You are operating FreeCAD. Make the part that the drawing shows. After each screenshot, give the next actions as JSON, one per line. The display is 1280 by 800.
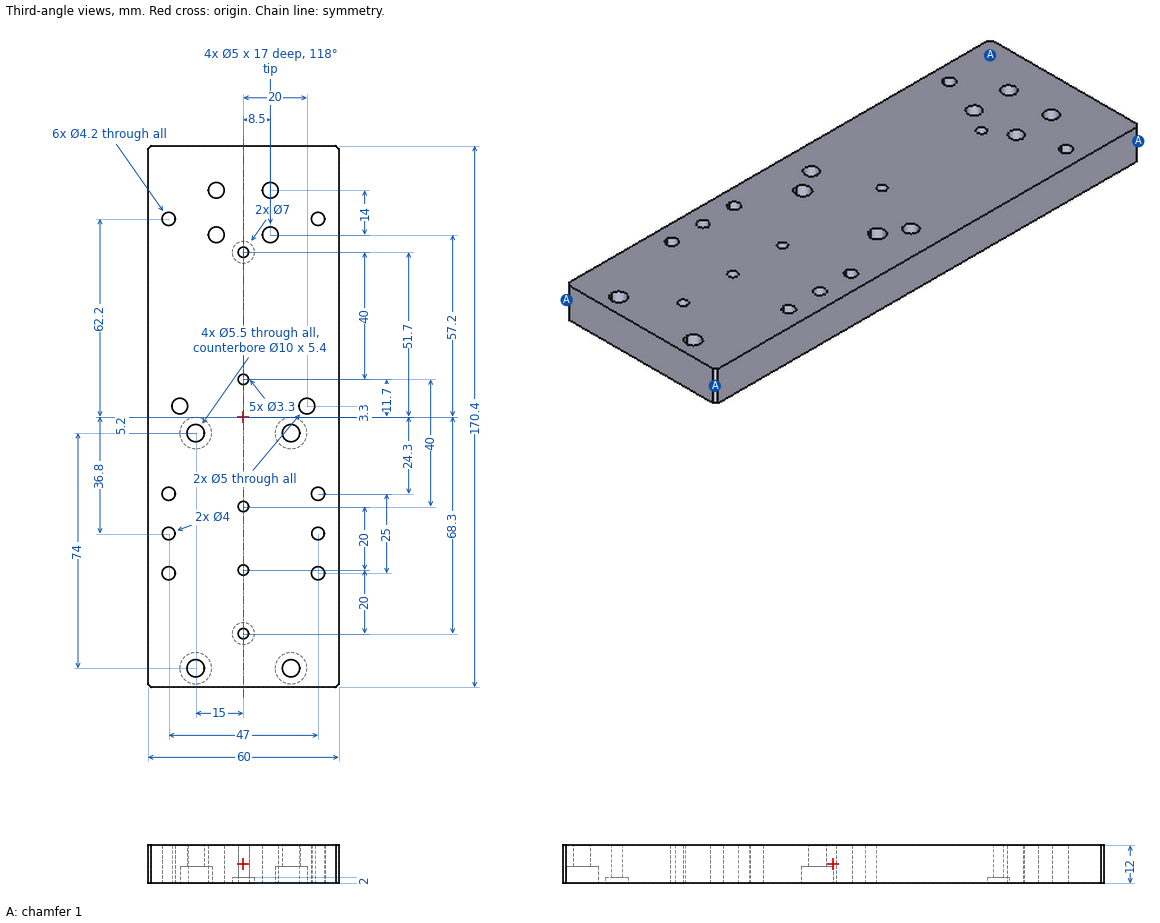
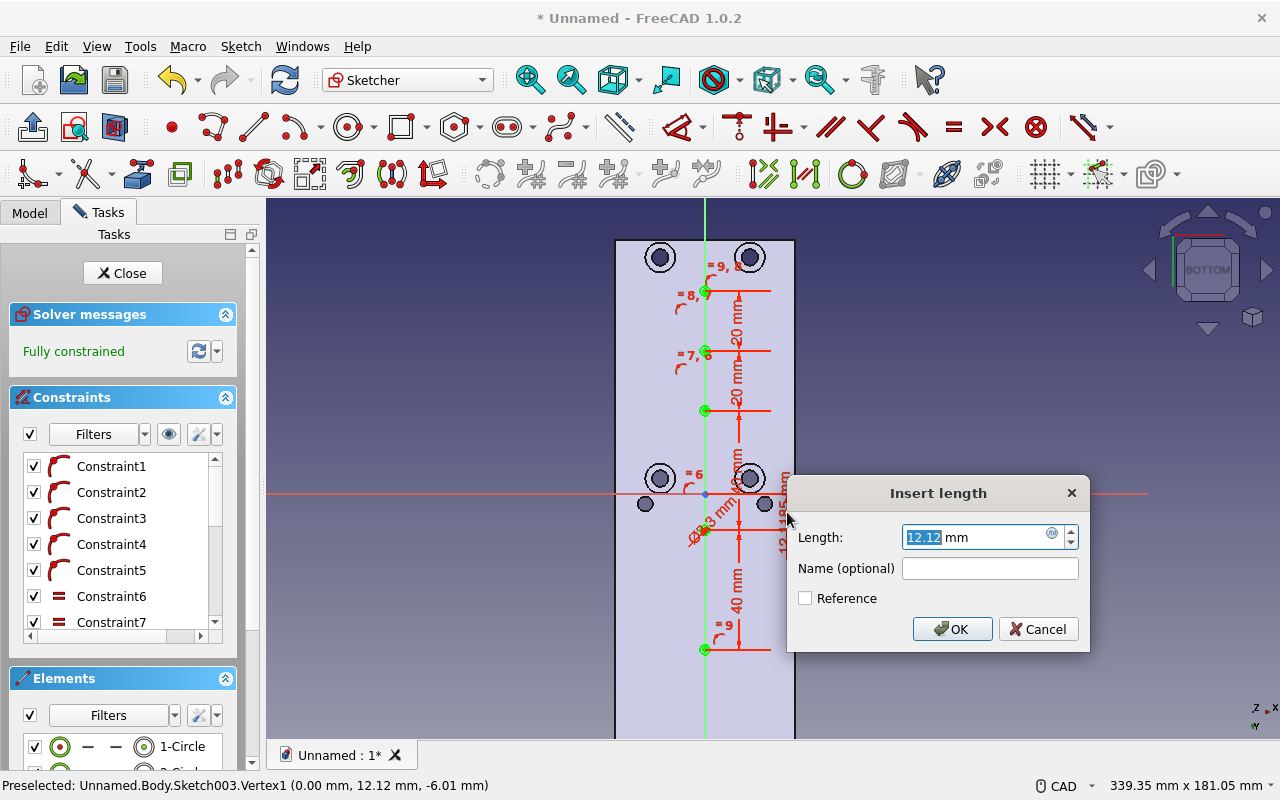
{"action": "type", "text": "11.7"}
{"action": "key", "text": "Return"}
{"action": "key", "text": "Escape"}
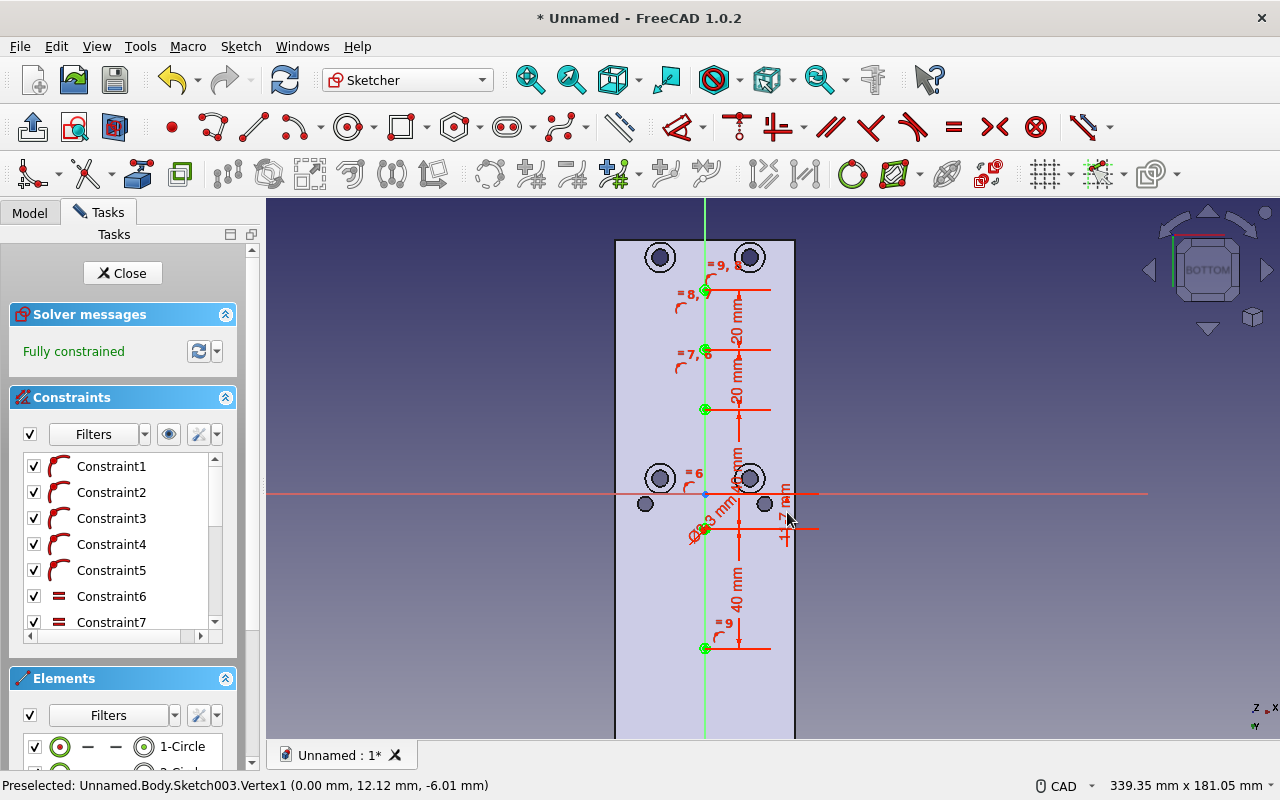
{"action": "left_click", "coordinate": [123, 273]}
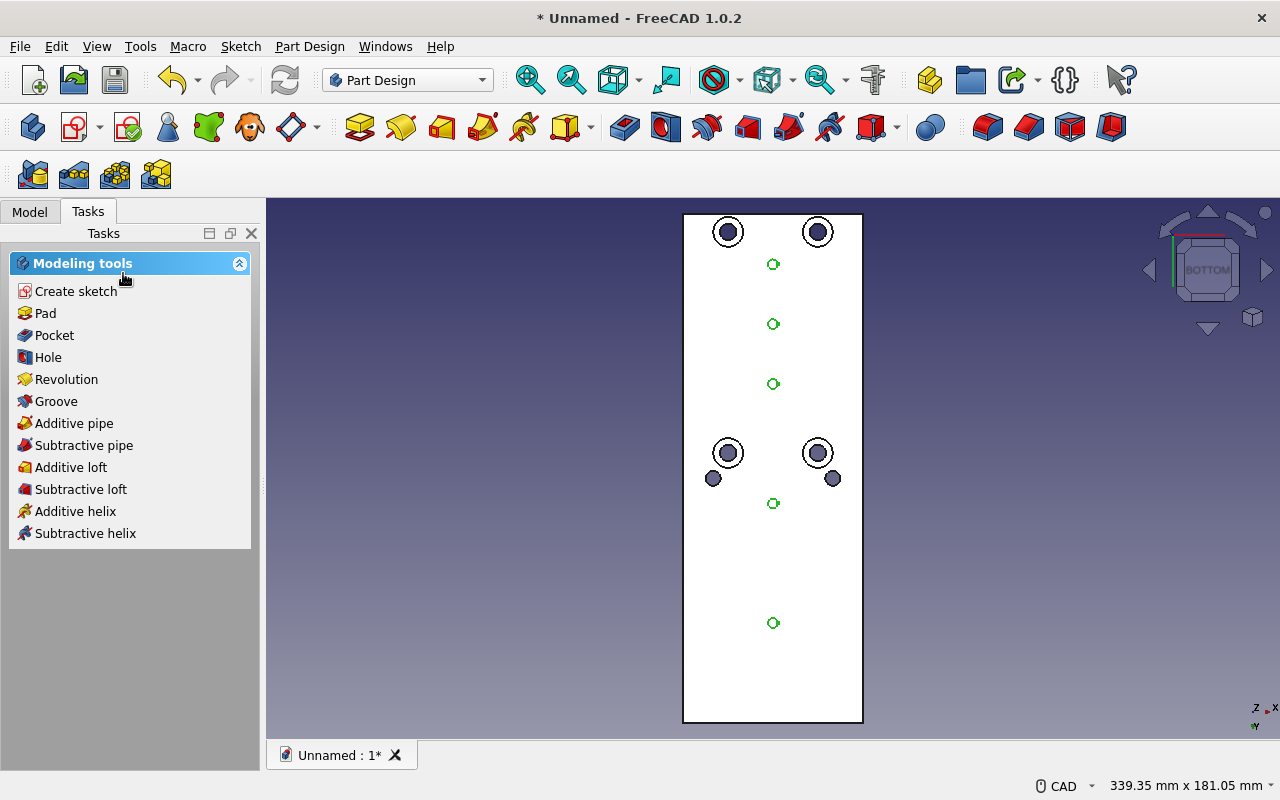
{"action": "left_click", "coordinate": [625, 128]}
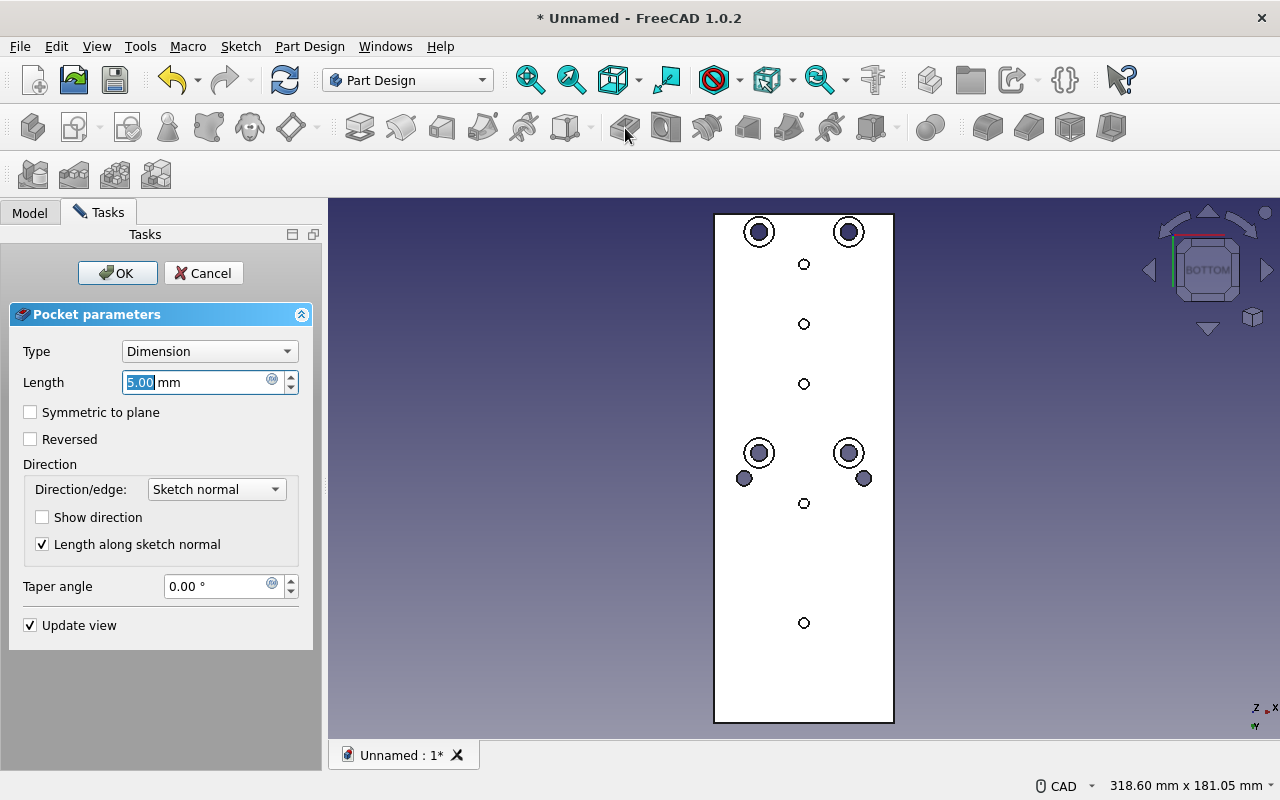
{"action": "left_click", "coordinate": [210, 352]}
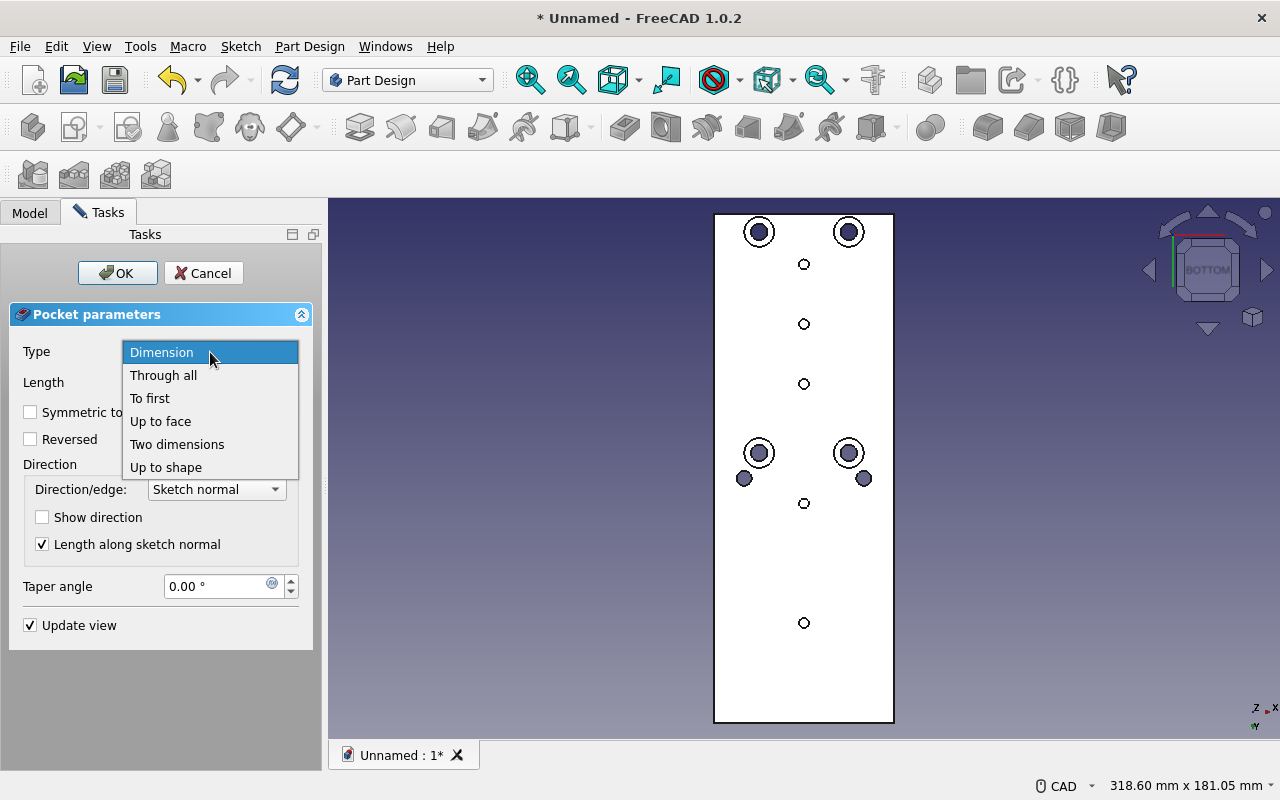
{"action": "left_click", "coordinate": [208, 376]}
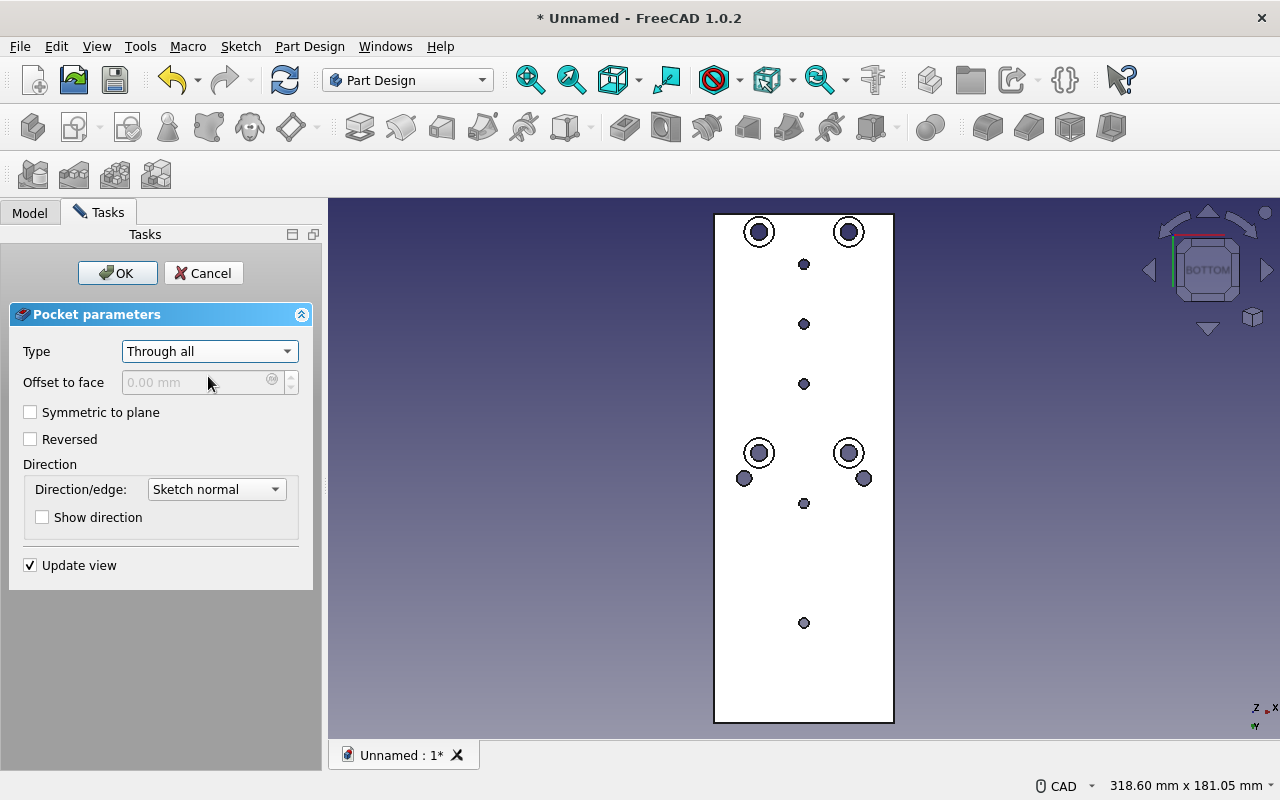
{"action": "left_click", "coordinate": [118, 273]}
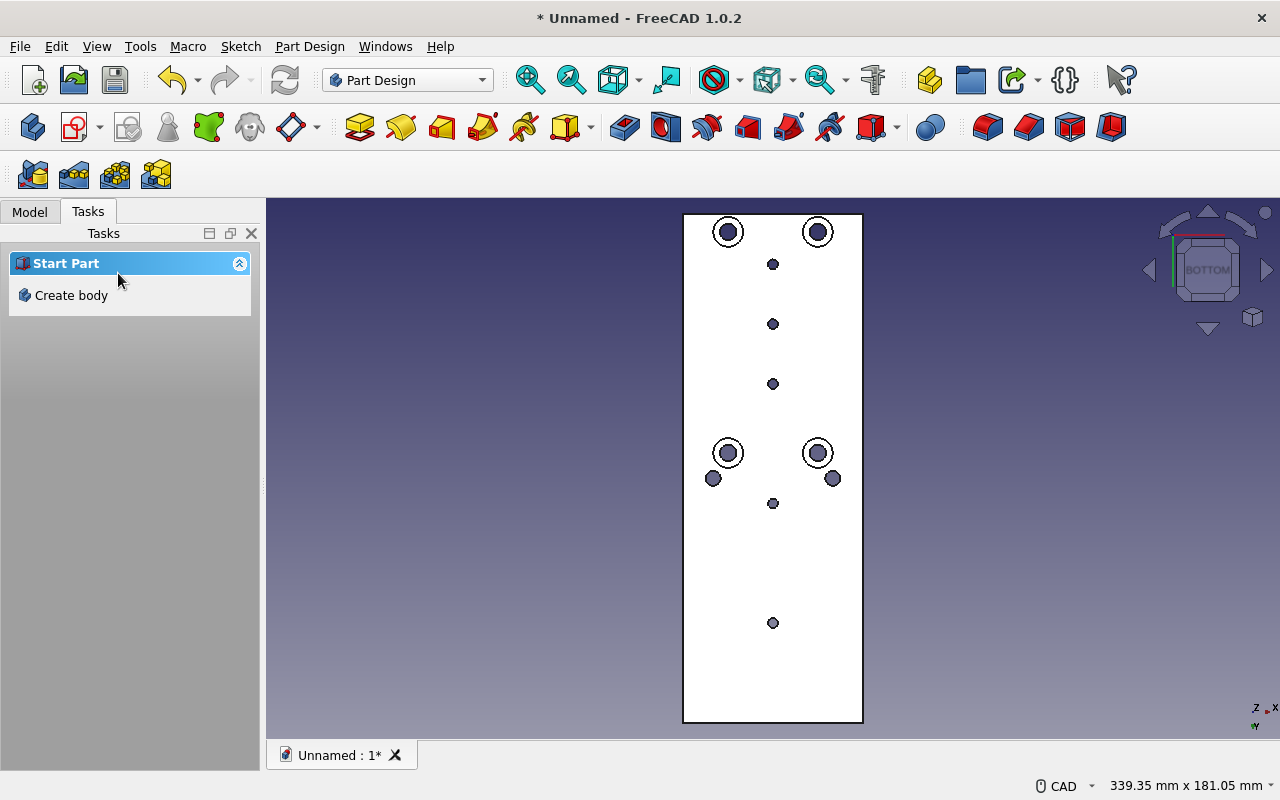
{"action": "left_click", "coordinate": [747, 540]}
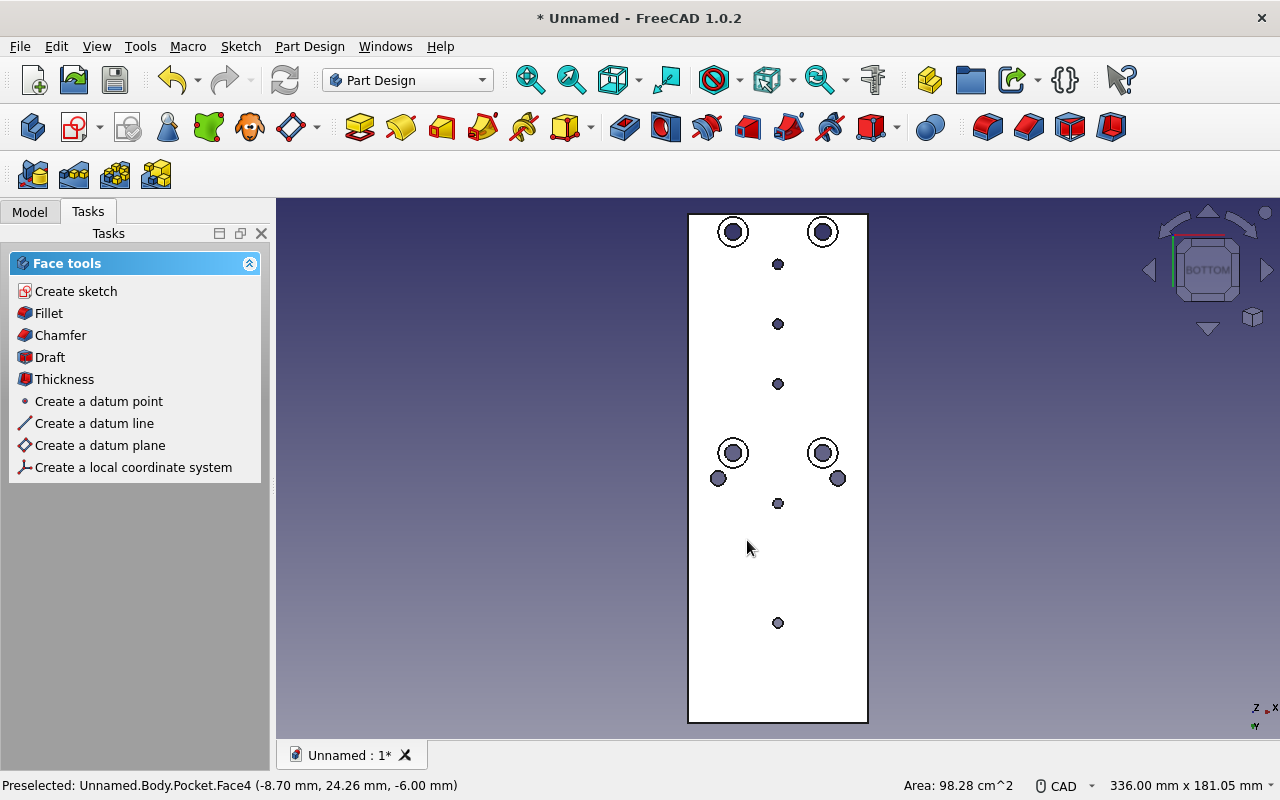
{"action": "left_click", "coordinate": [74, 128]}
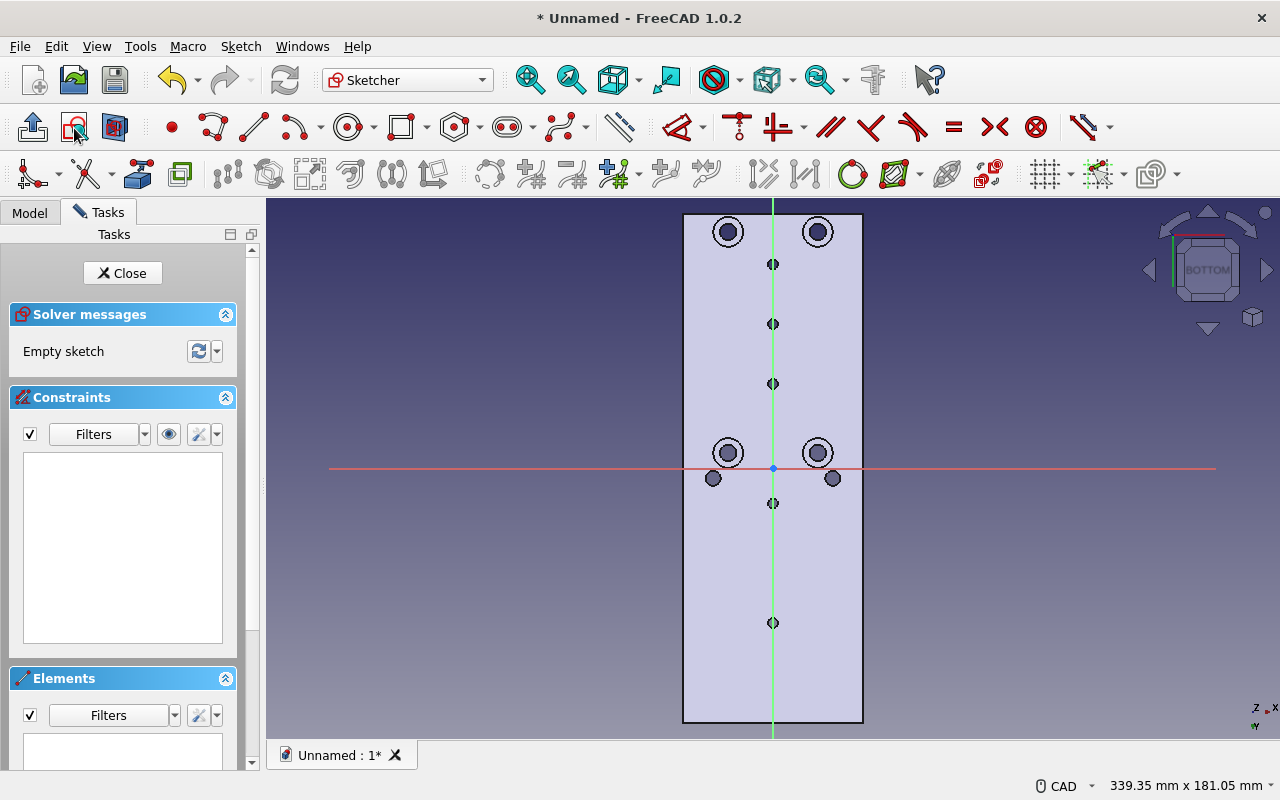
{"action": "left_click", "coordinate": [348, 128]}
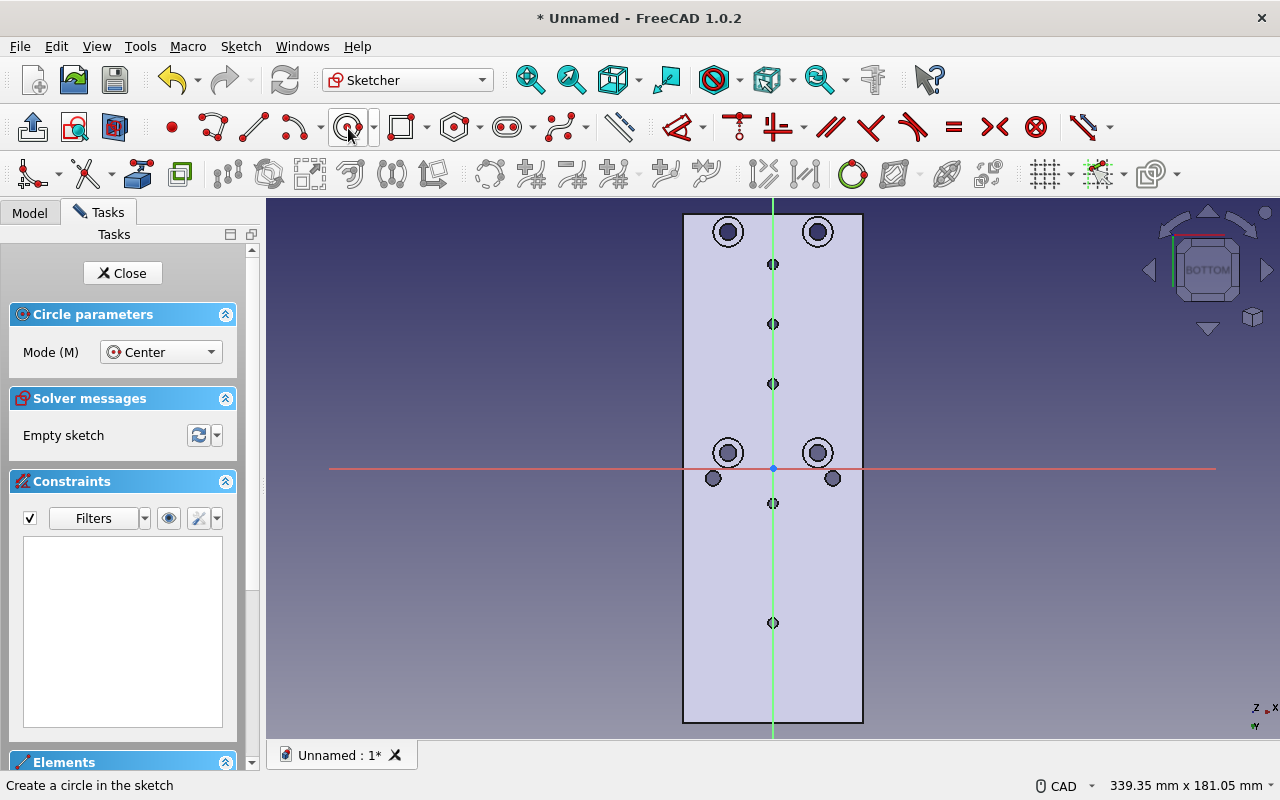
{"action": "scroll", "coordinate": [773, 623], "scroll_direction": "up", "scroll_amount": 4}